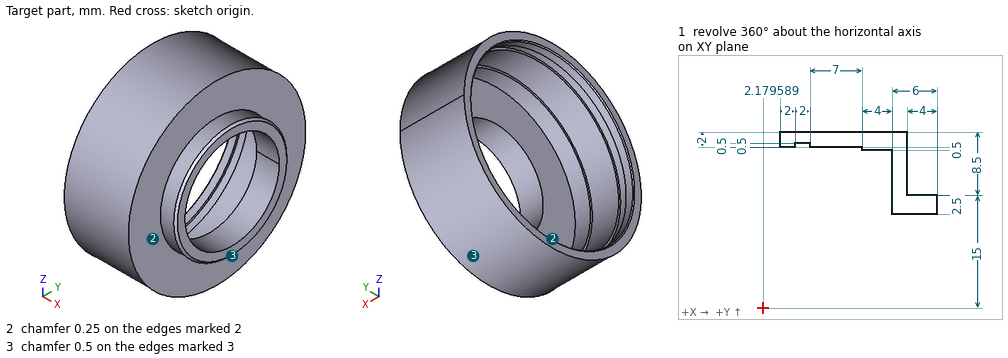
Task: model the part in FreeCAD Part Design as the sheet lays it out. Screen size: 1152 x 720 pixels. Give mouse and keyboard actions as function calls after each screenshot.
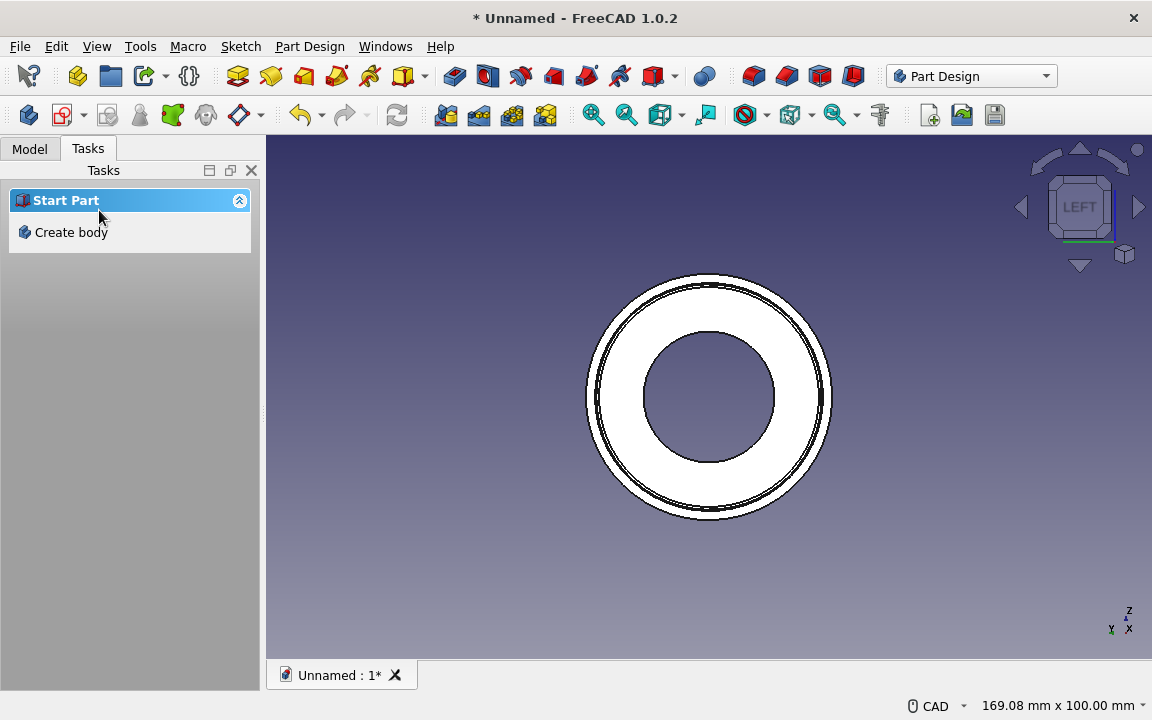
key(0)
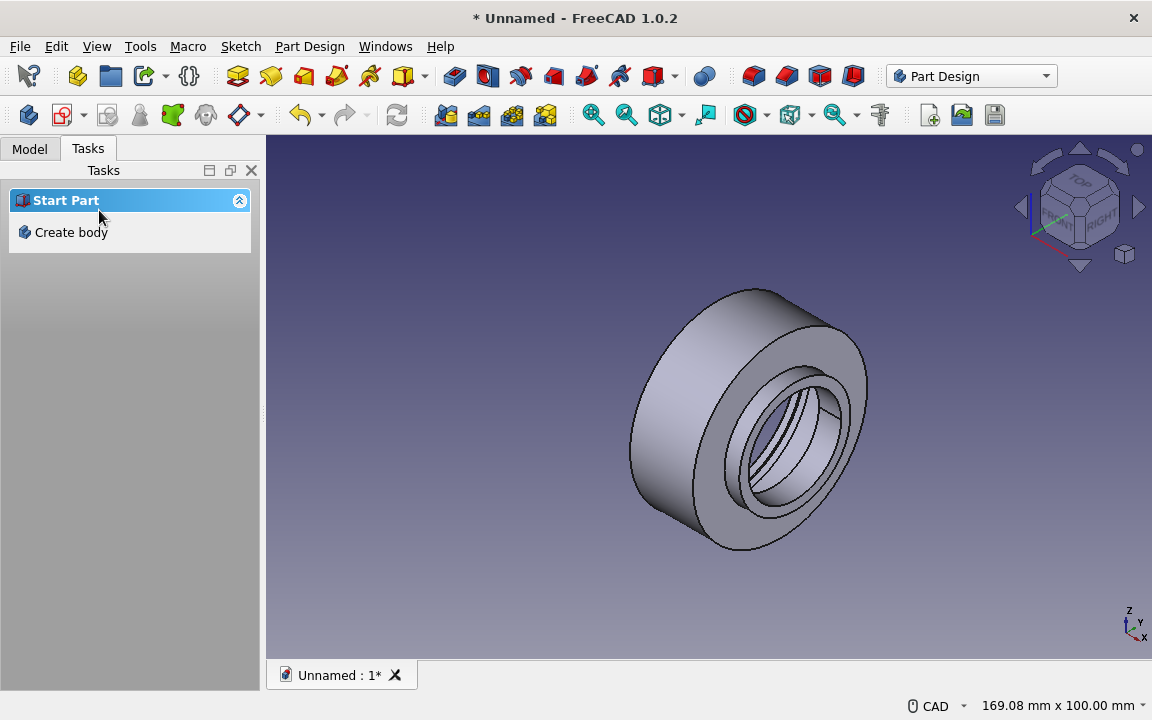
click(739, 478)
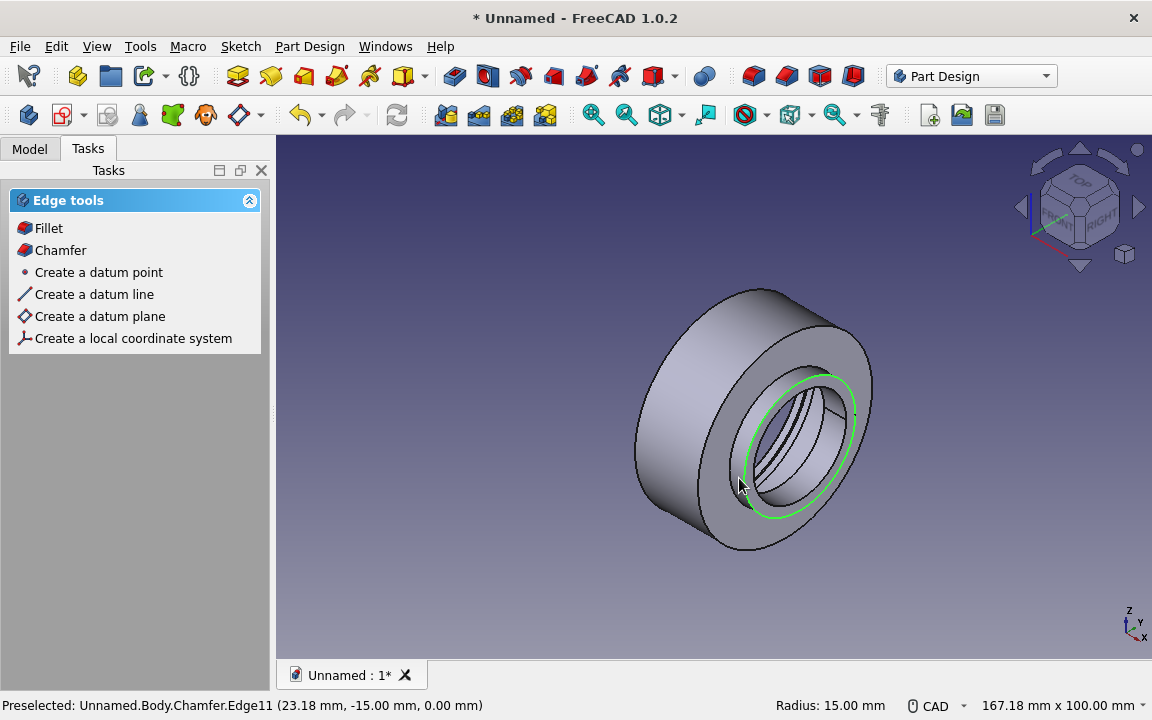
click(787, 76)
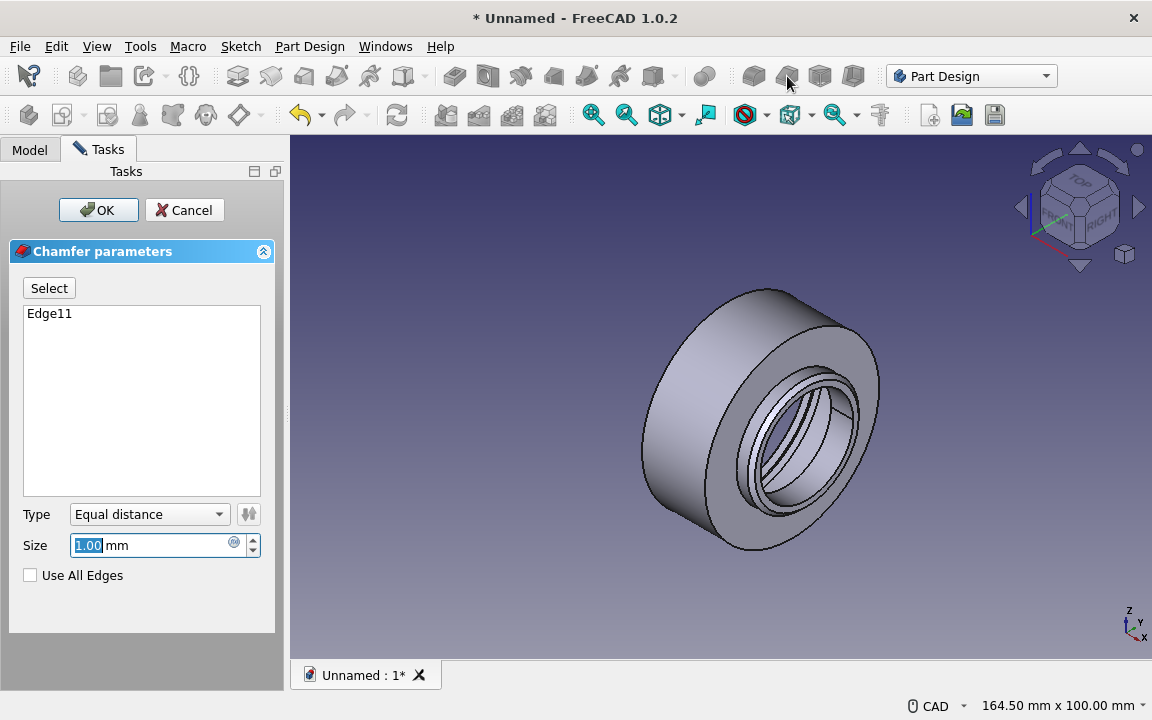
text(0.5)
key(Tab)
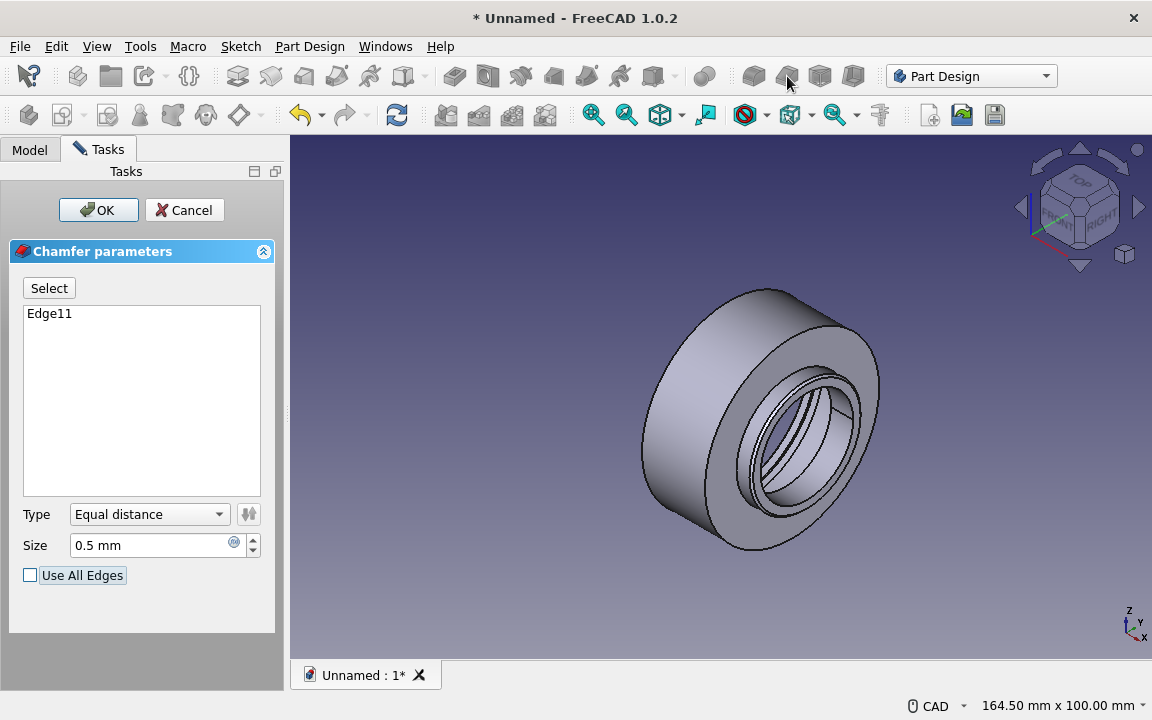
click(99, 210)